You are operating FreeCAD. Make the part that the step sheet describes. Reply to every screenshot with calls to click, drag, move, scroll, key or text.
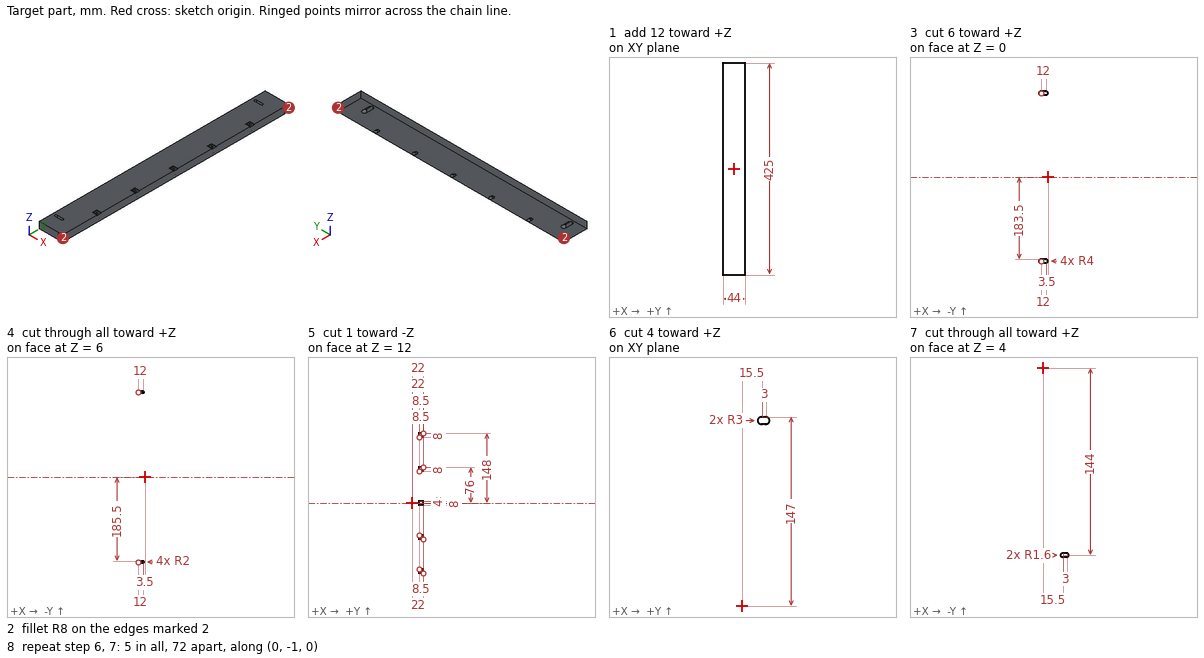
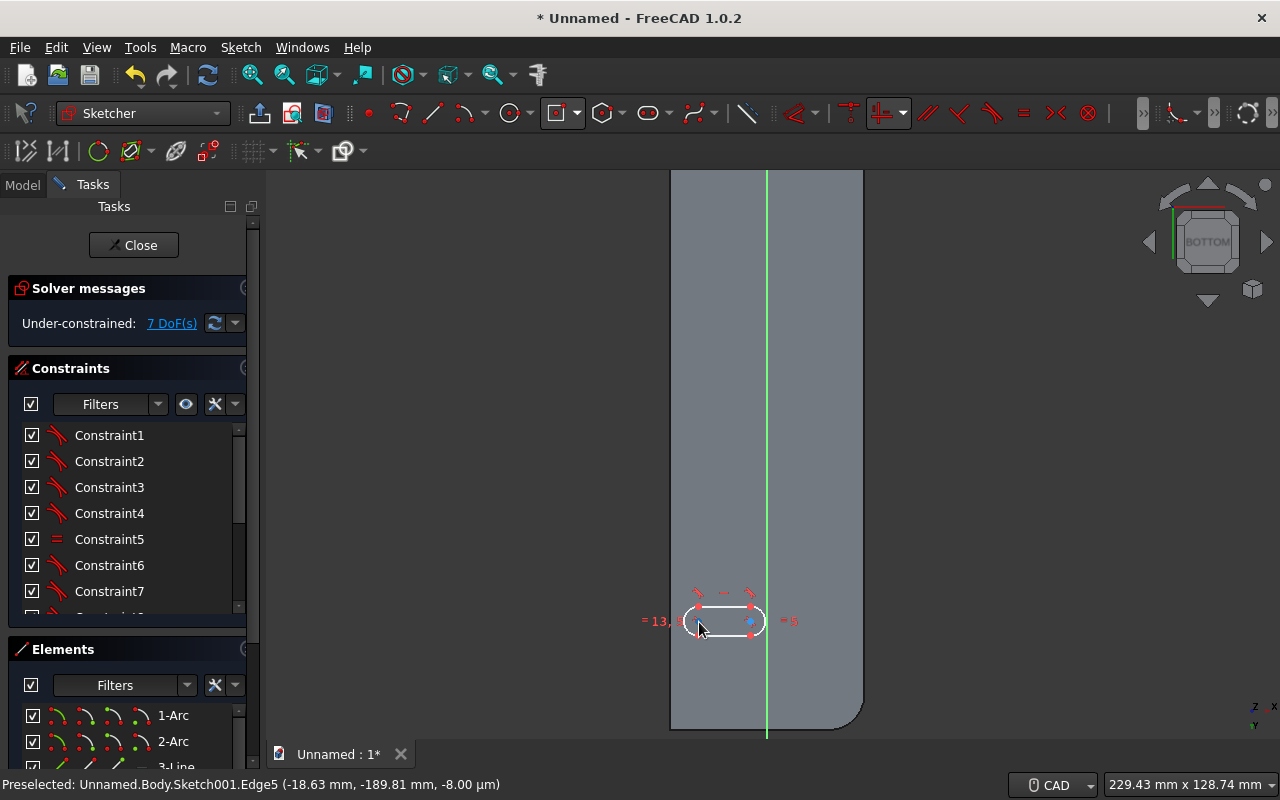
click(699, 621)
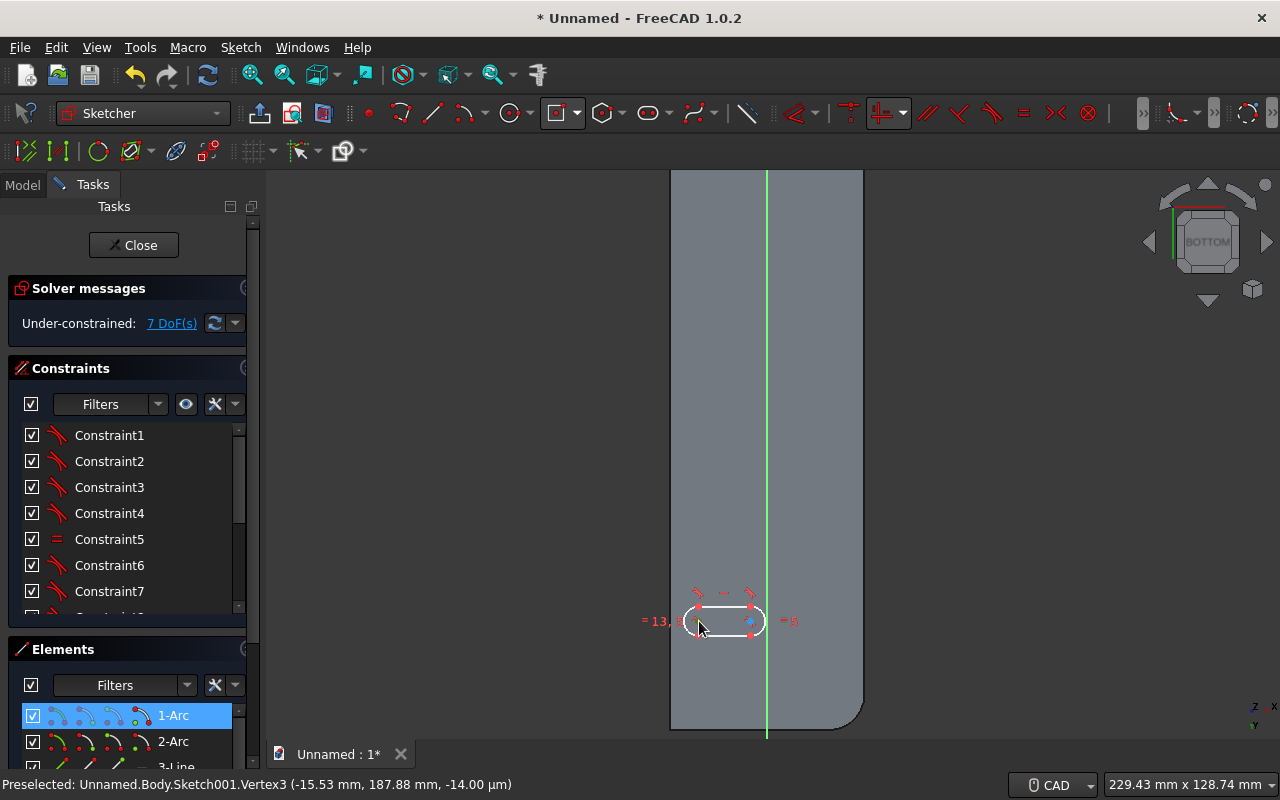
scroll(699, 622, down, 8)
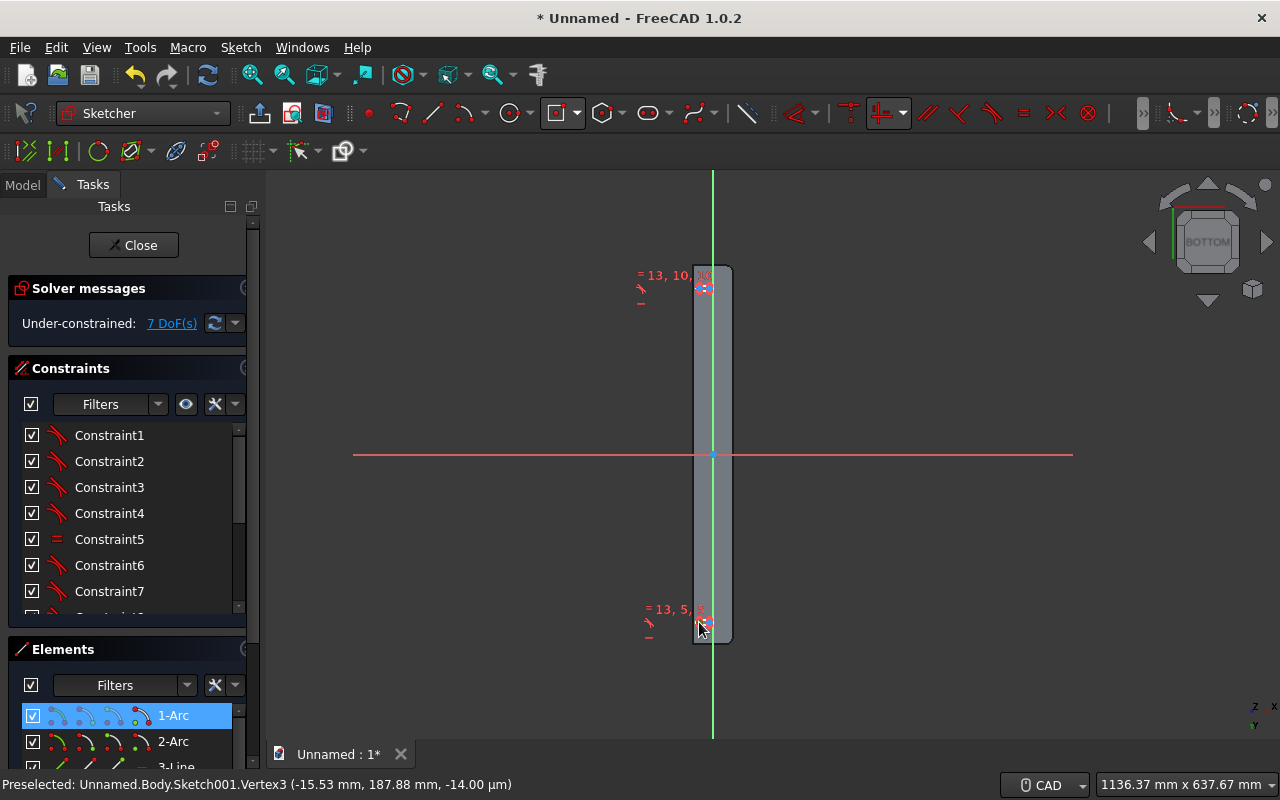
scroll(699, 289, up, 8)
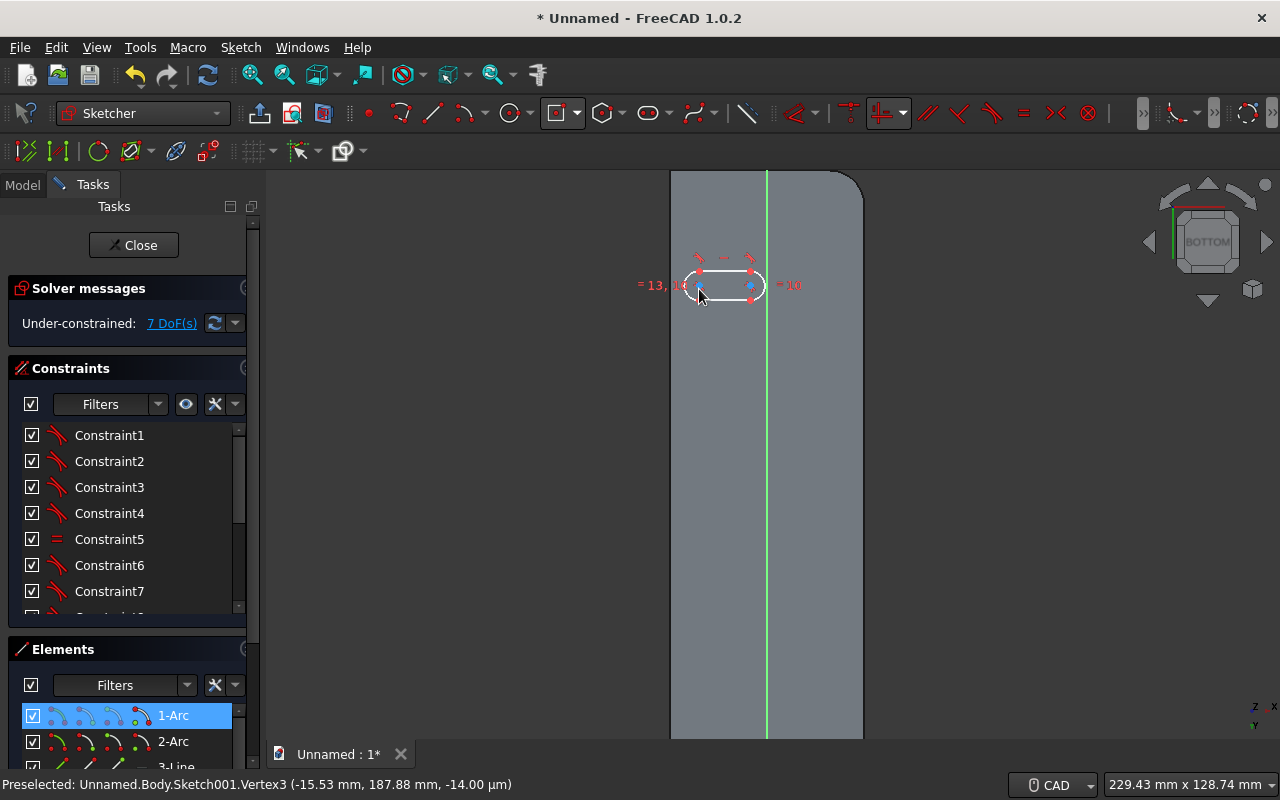
click(699, 286)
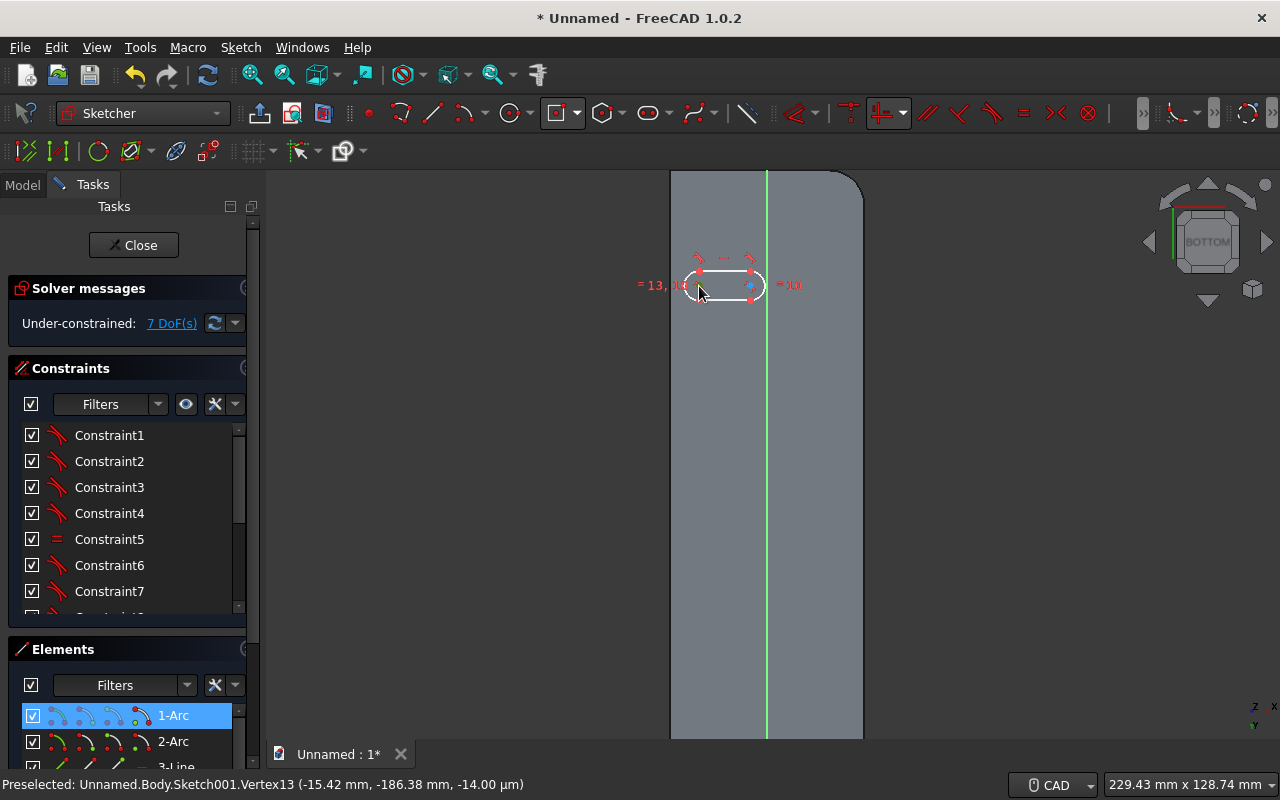
scroll(699, 289, down, 8)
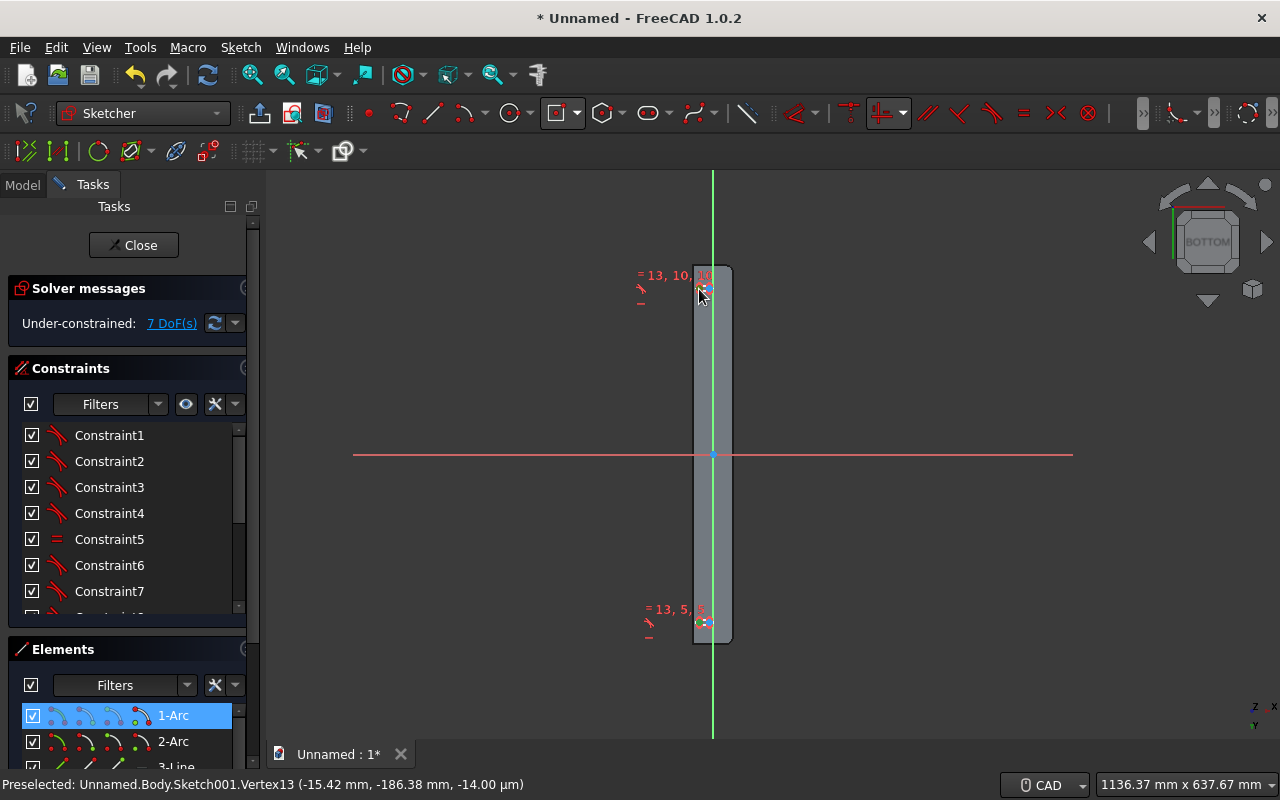
click(353, 455)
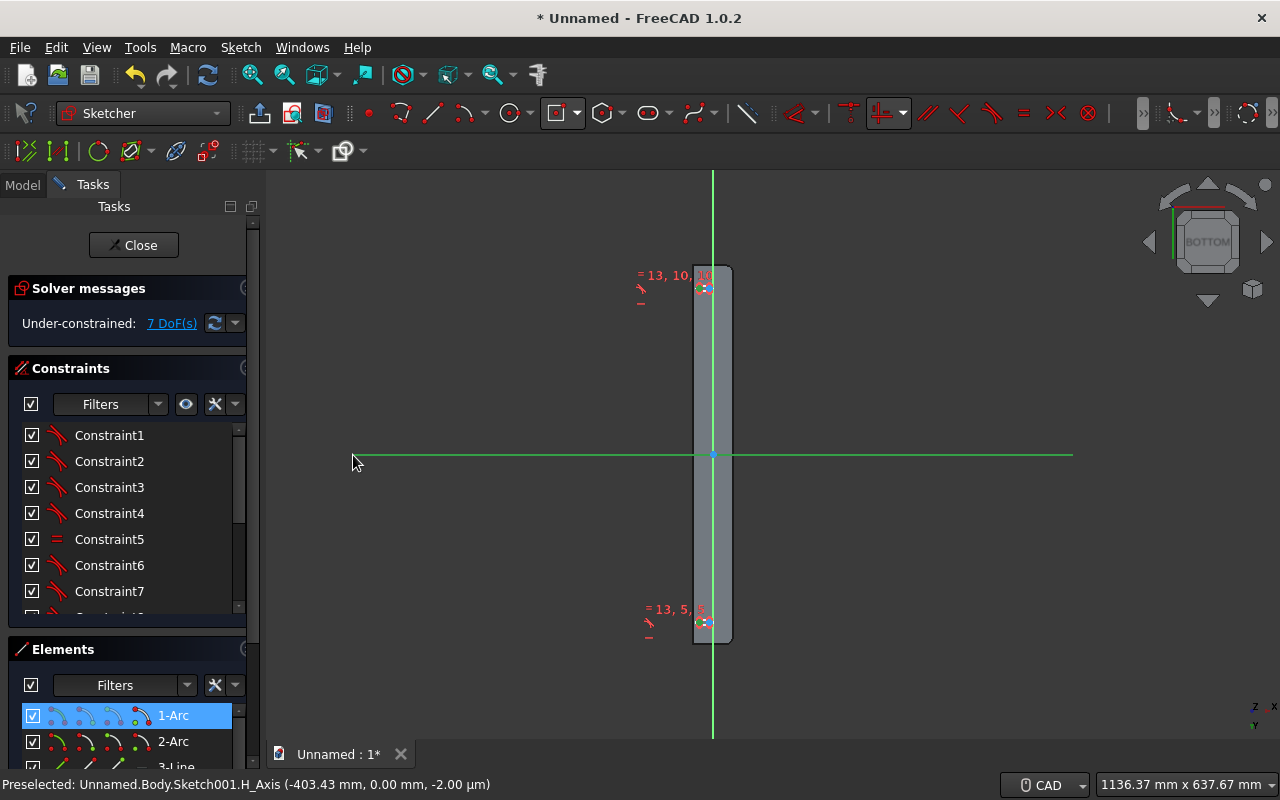
key(s)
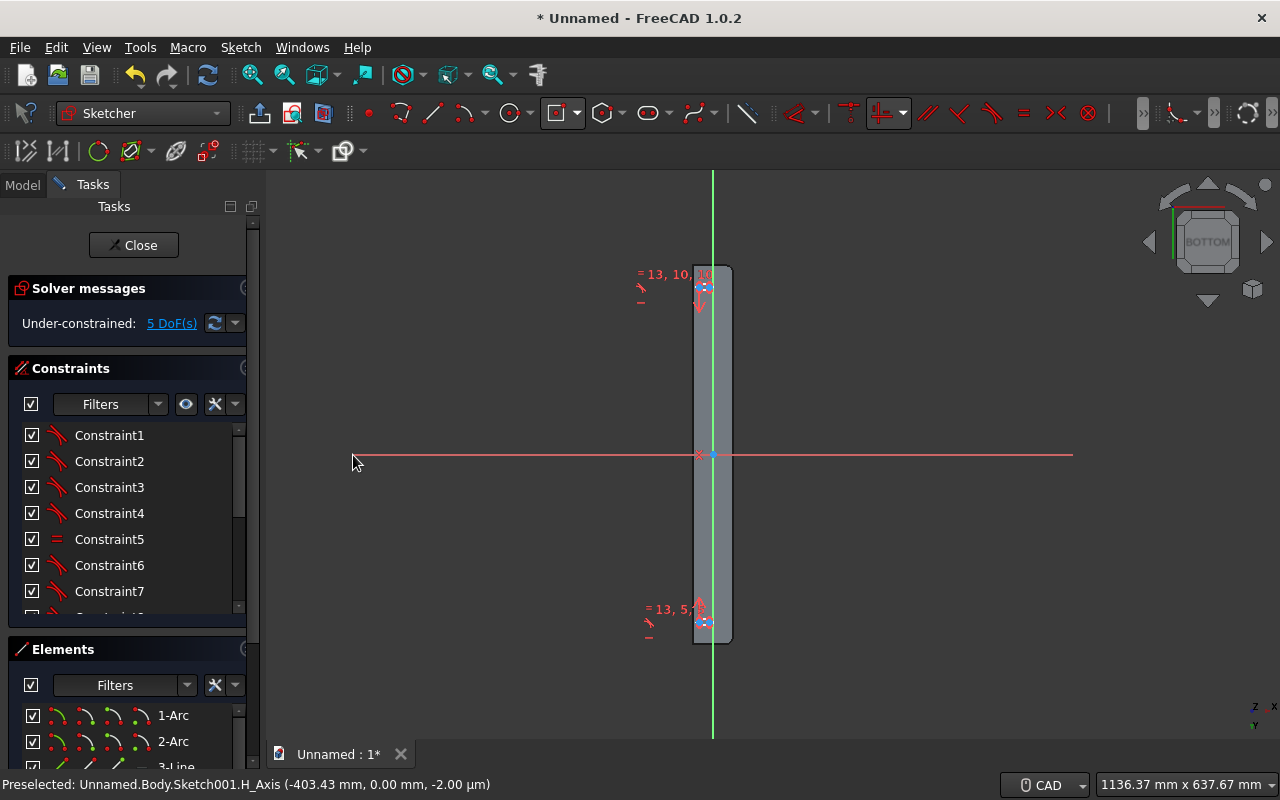
click(794, 114)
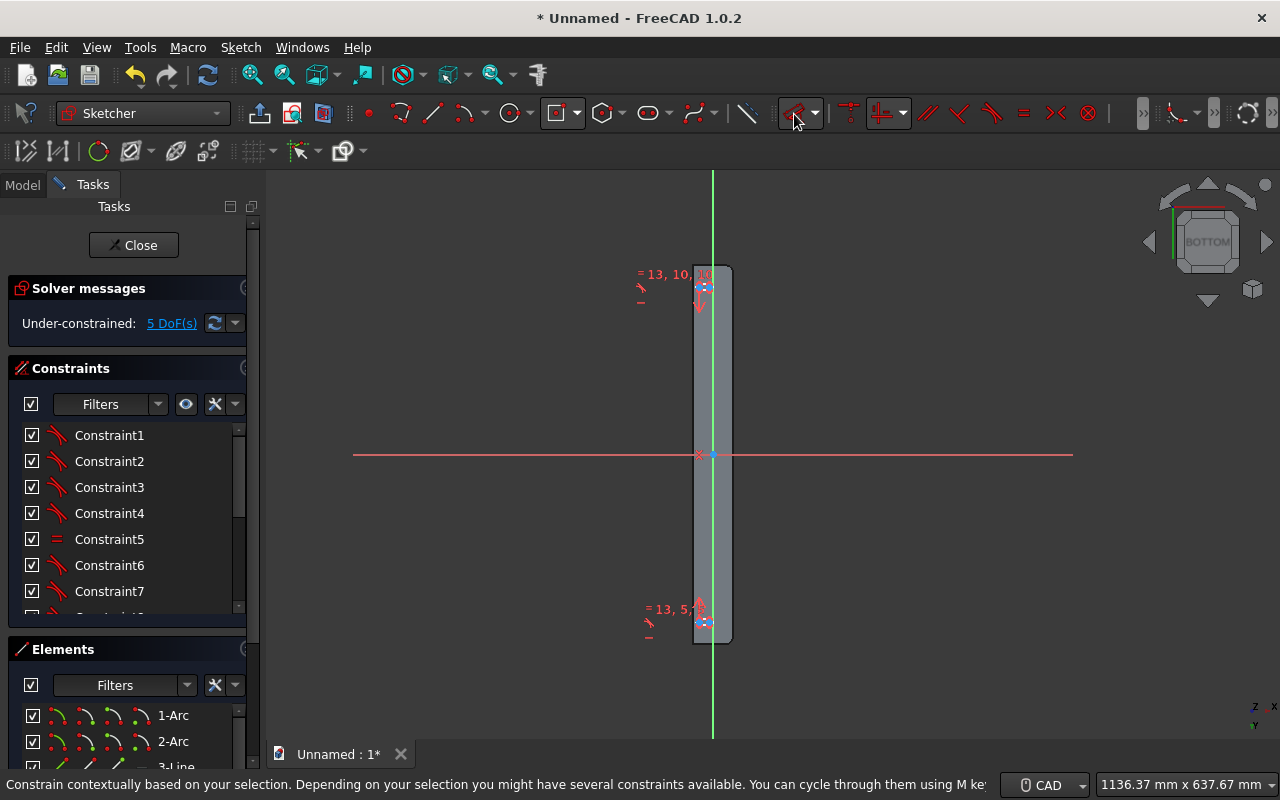
scroll(696, 622, up, 13)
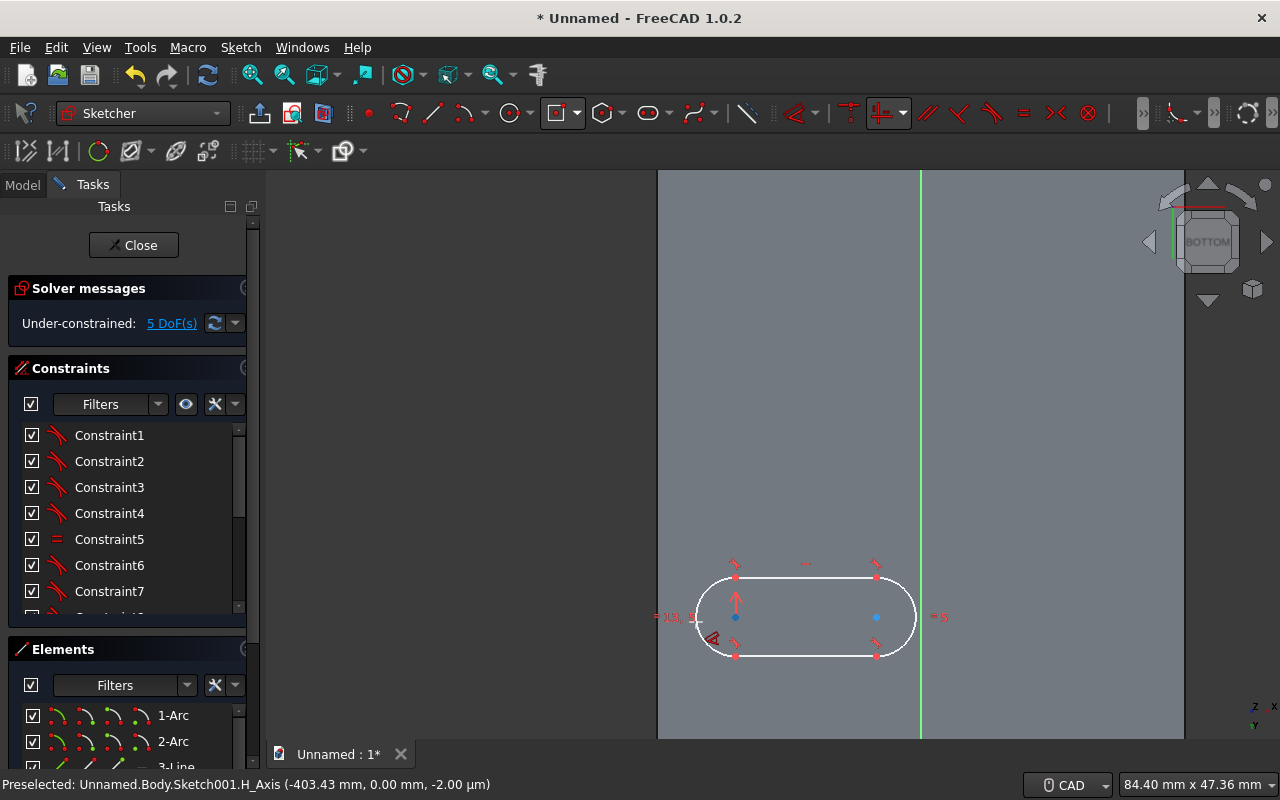
click(696, 617)
click(664, 617)